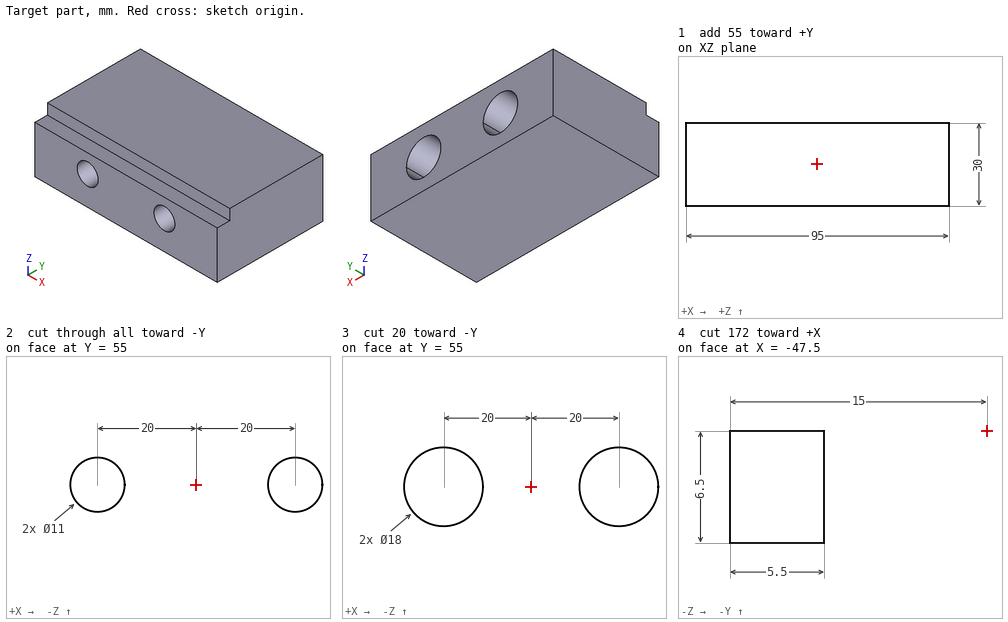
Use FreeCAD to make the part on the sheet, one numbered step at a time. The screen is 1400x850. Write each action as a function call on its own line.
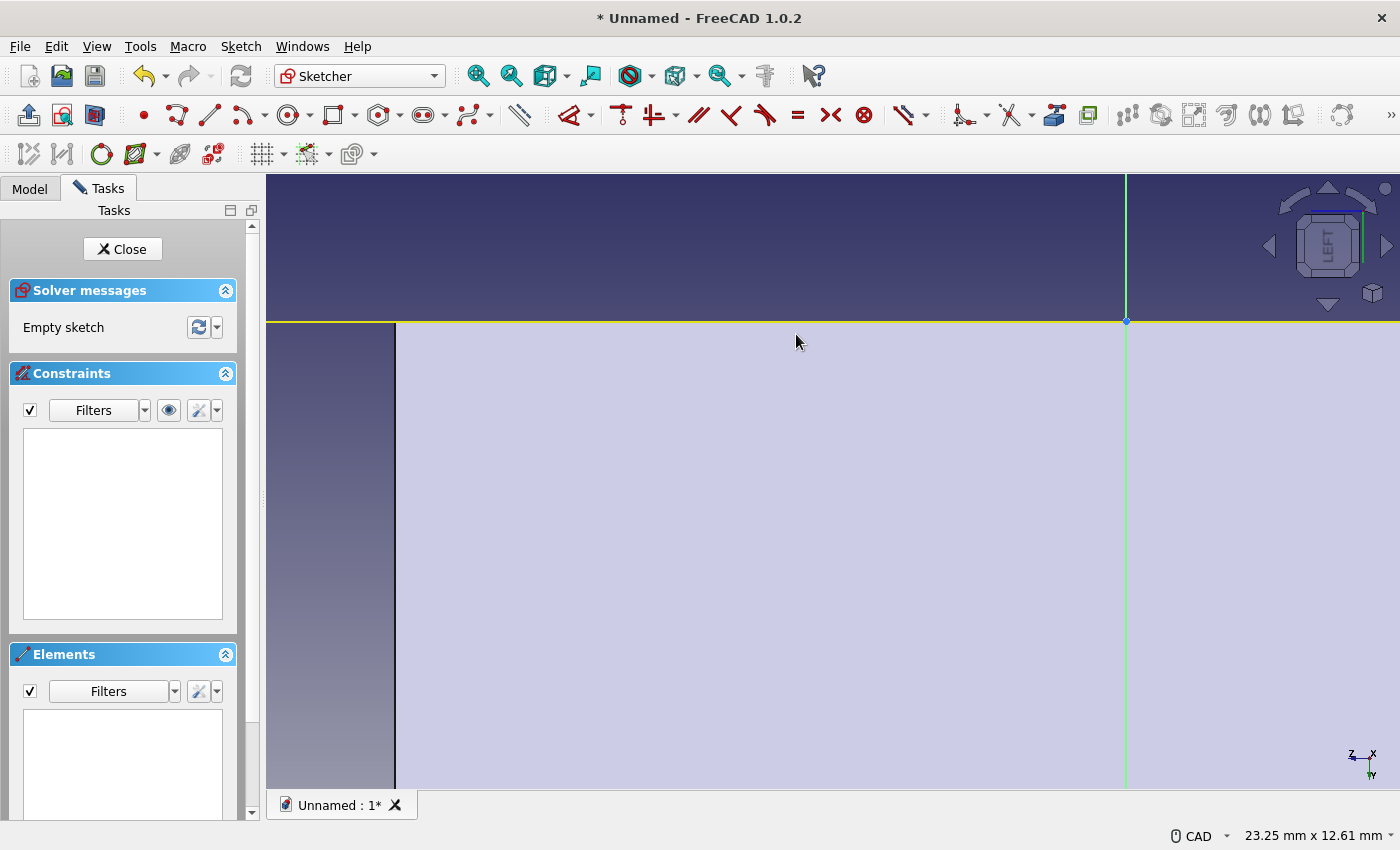
click(332, 116)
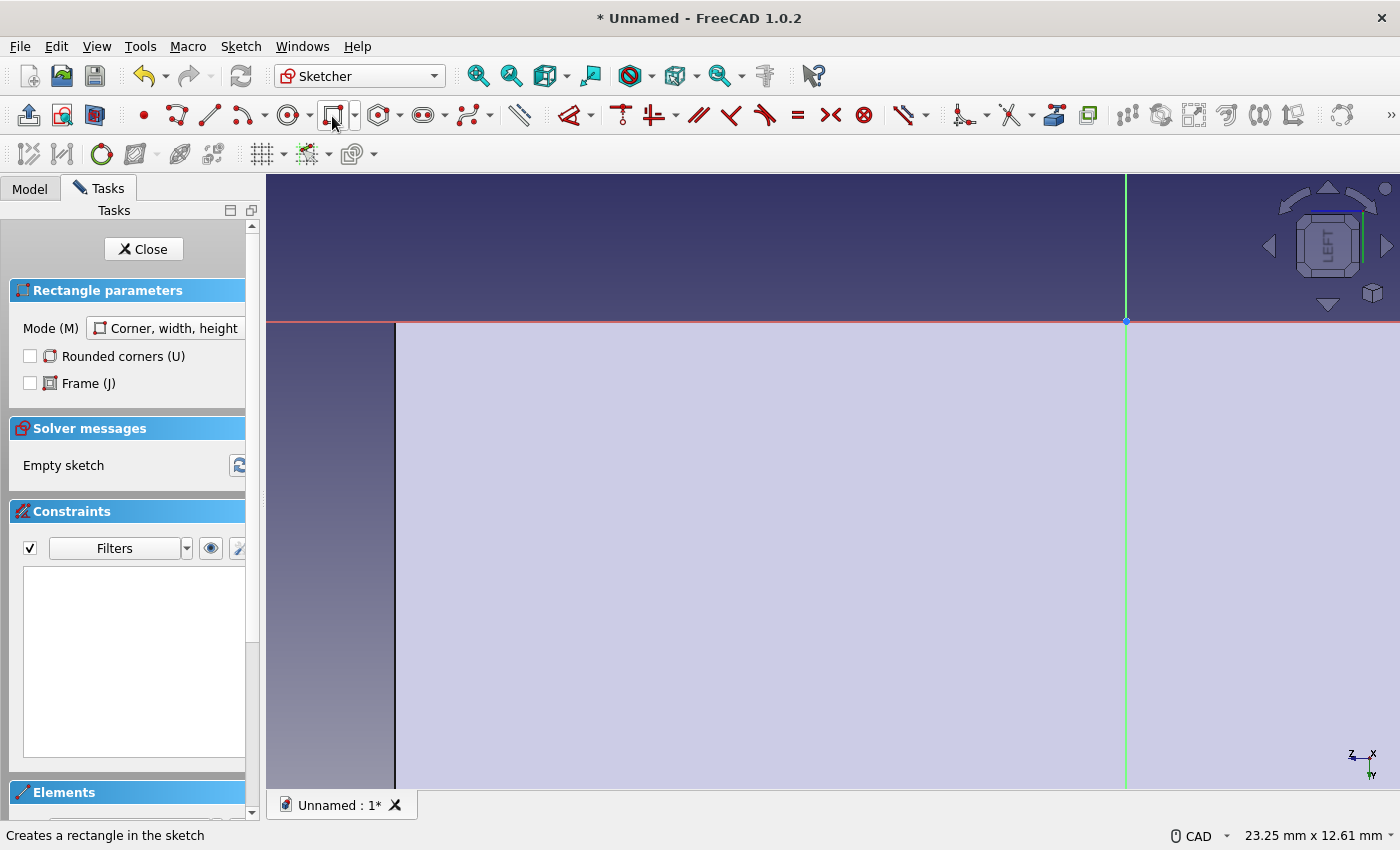
click(395, 322)
move(663, 639)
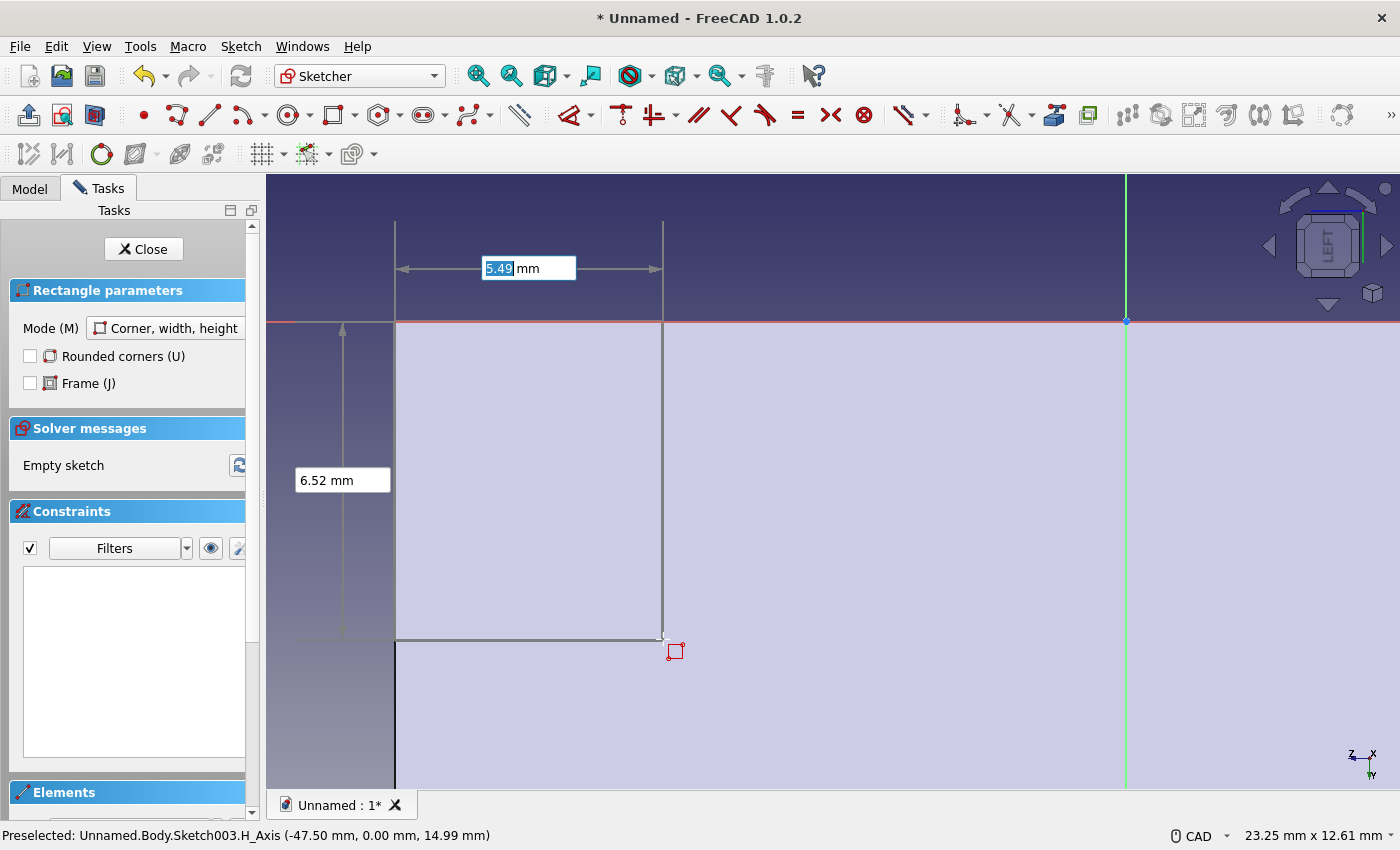
text(5.5)
key(Tab)
text(6.5)
key(Return)
key(Escape)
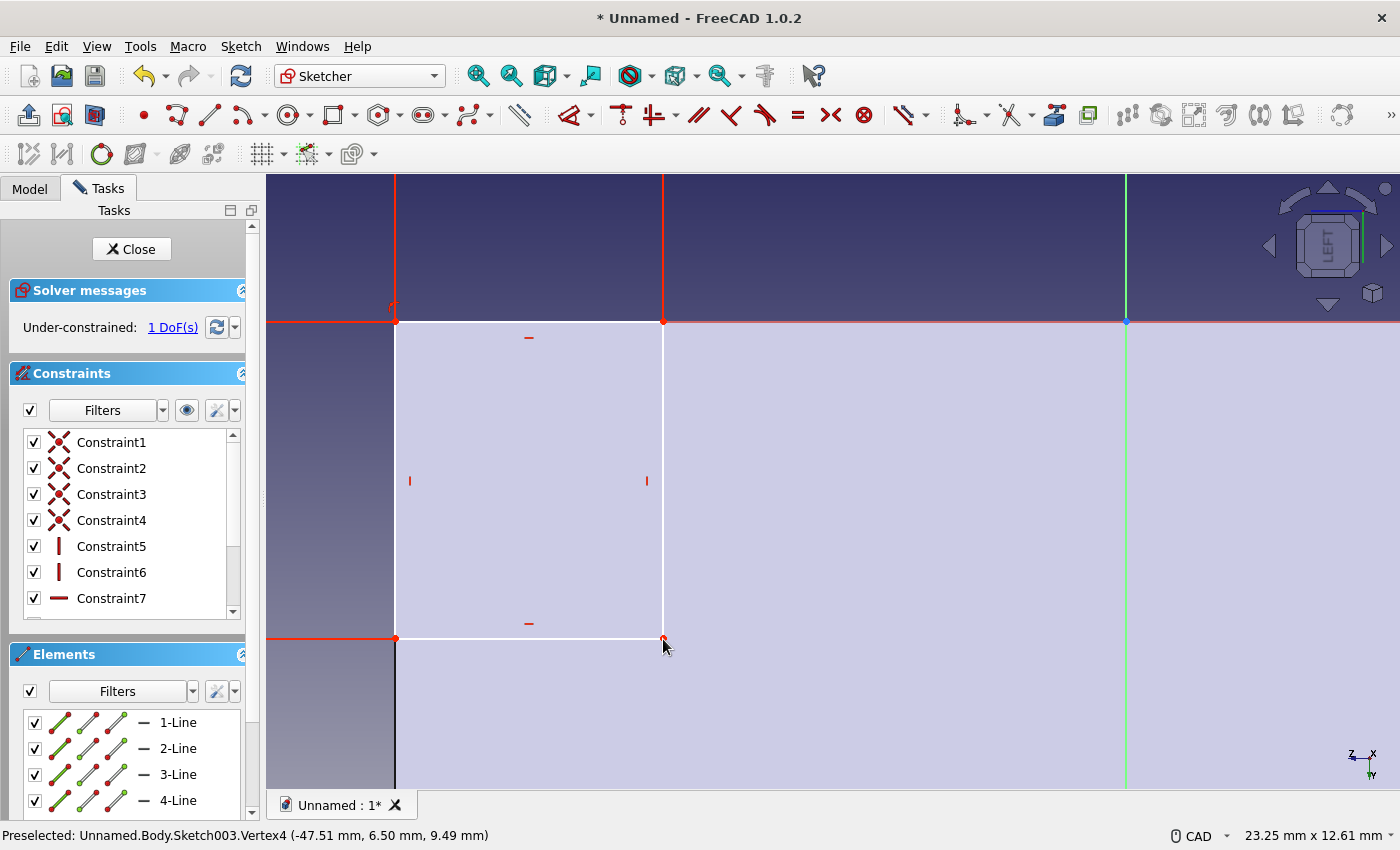
click(568, 116)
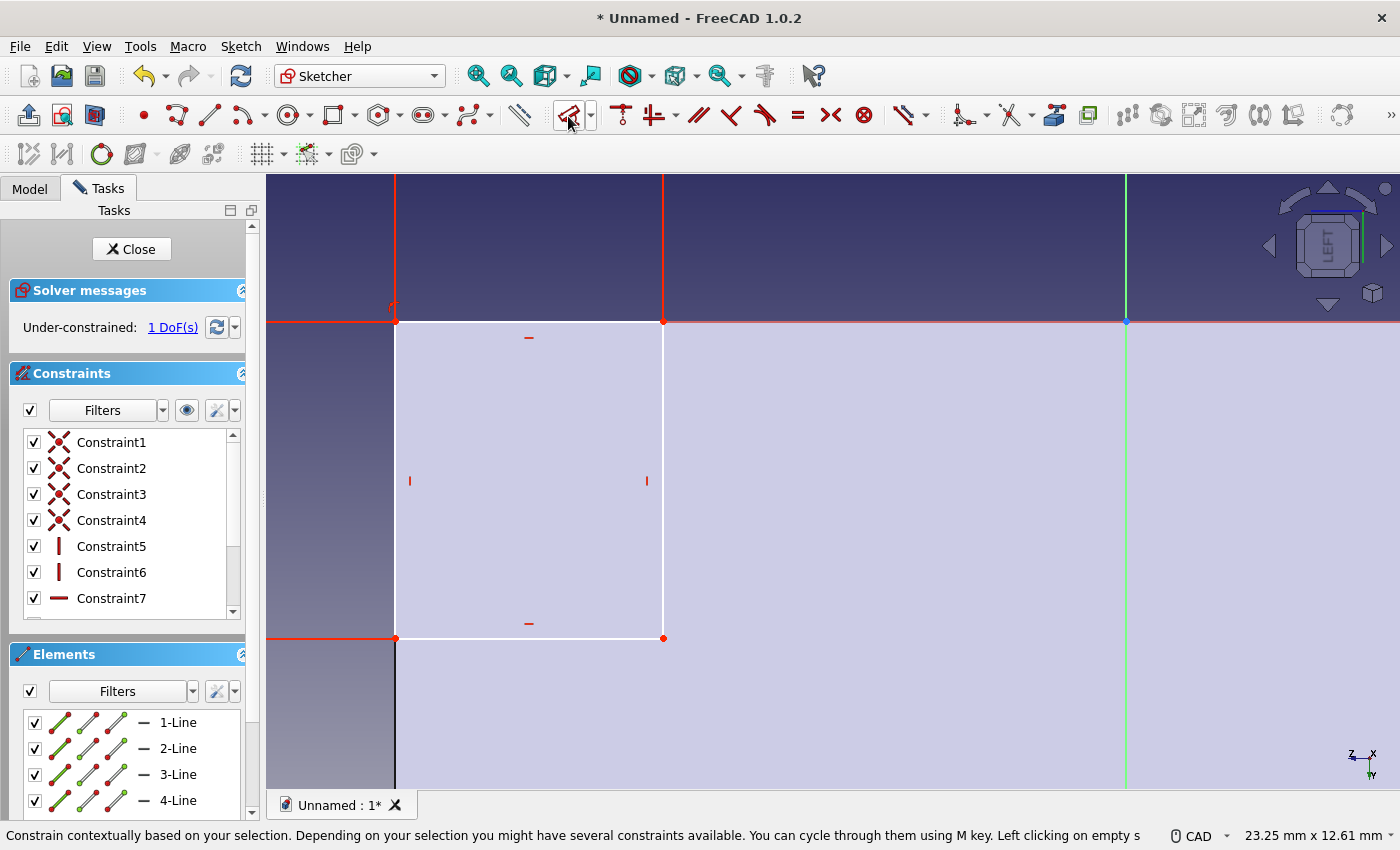
click(395, 322)
click(761, 288)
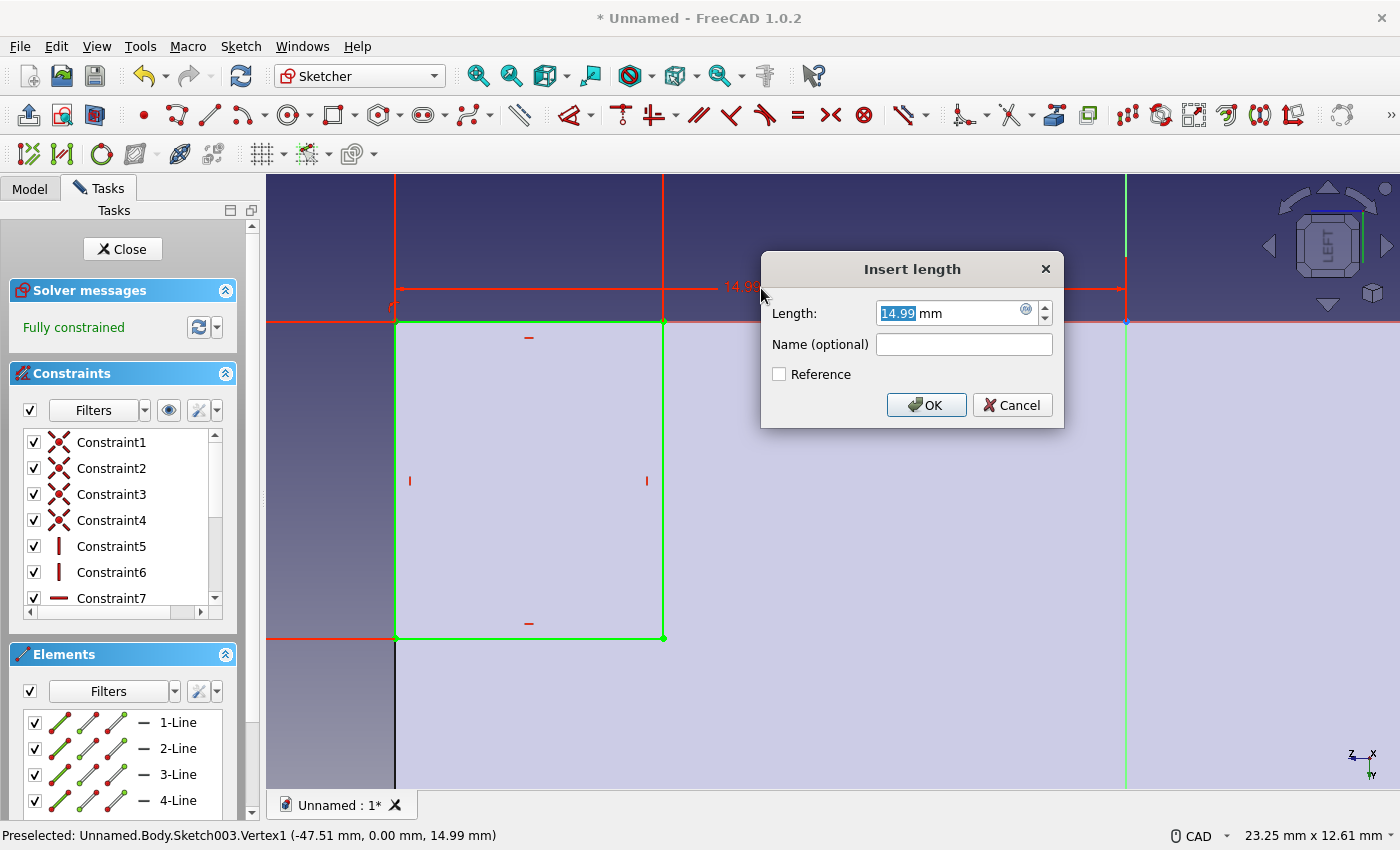
text(15)
key(Return)
key(Escape)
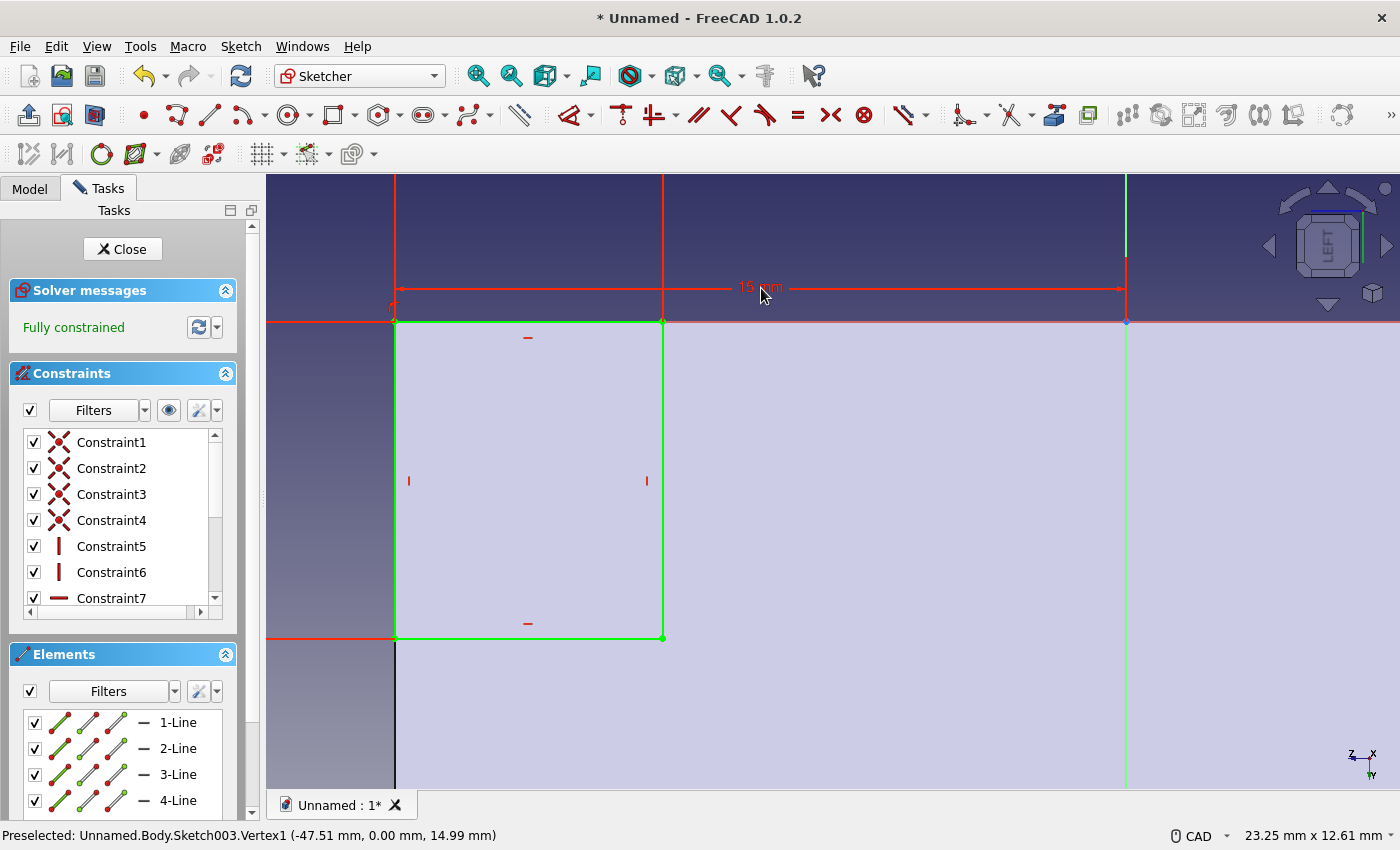
click(123, 249)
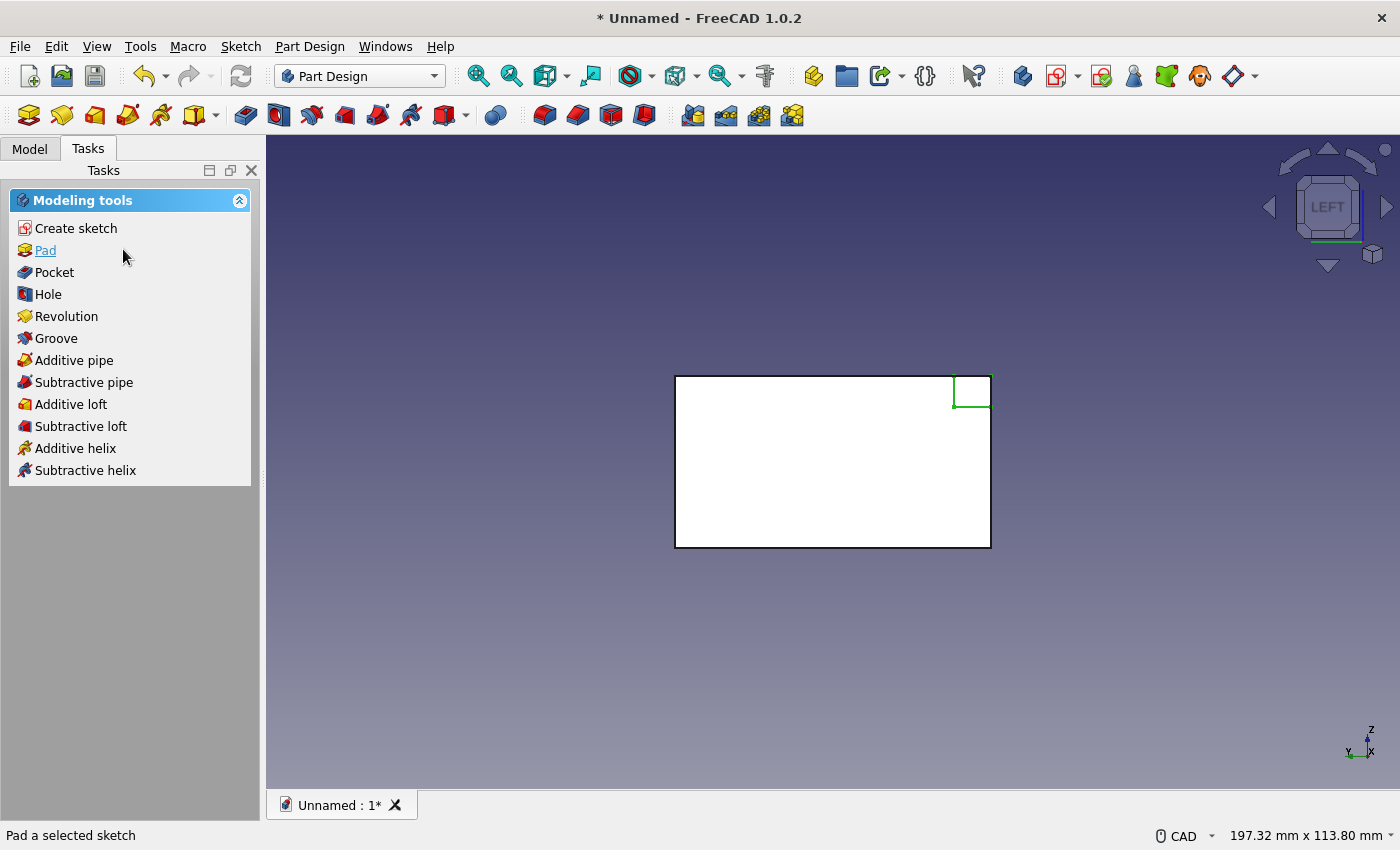
click(246, 116)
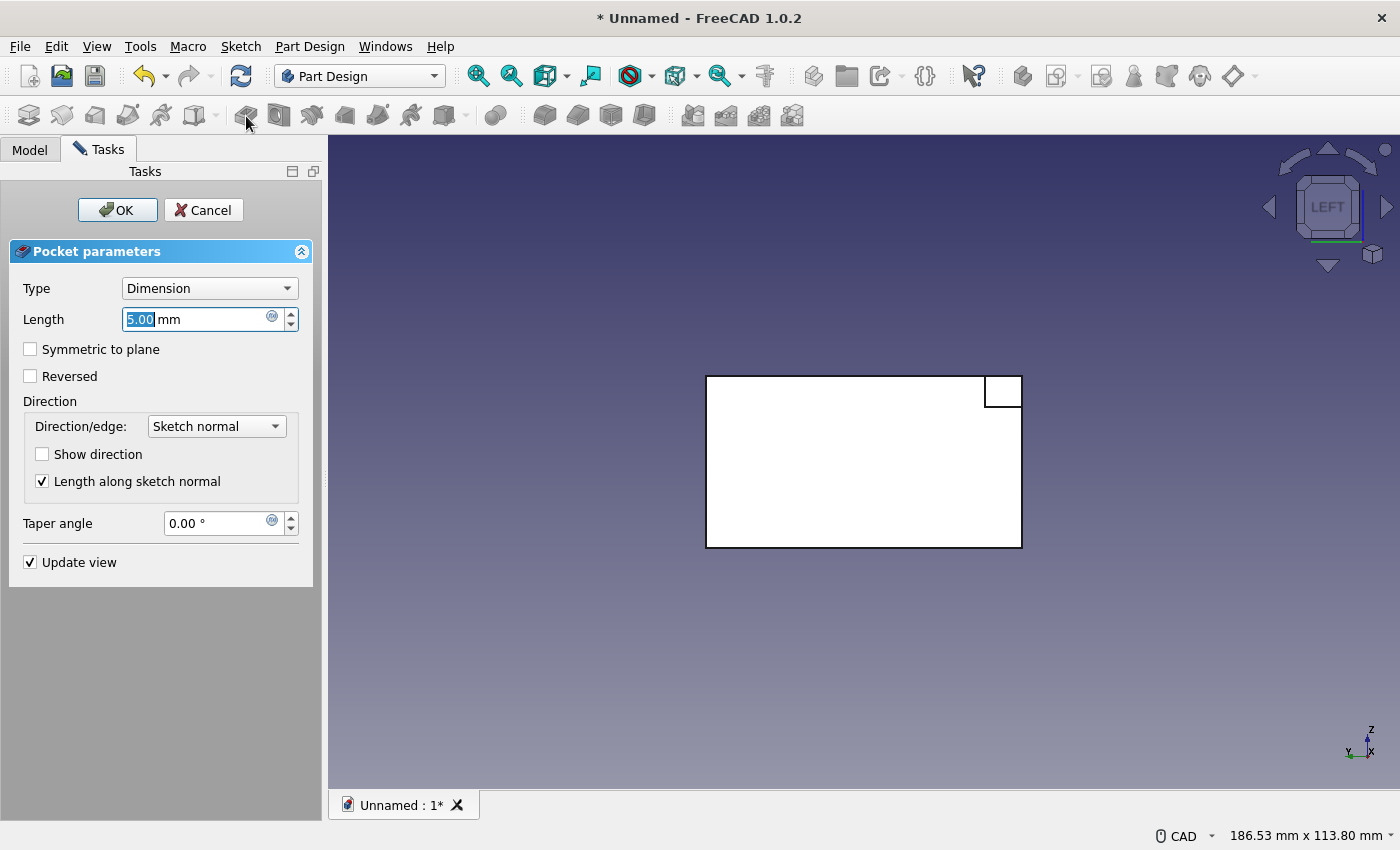
text(172)
key(Tab)